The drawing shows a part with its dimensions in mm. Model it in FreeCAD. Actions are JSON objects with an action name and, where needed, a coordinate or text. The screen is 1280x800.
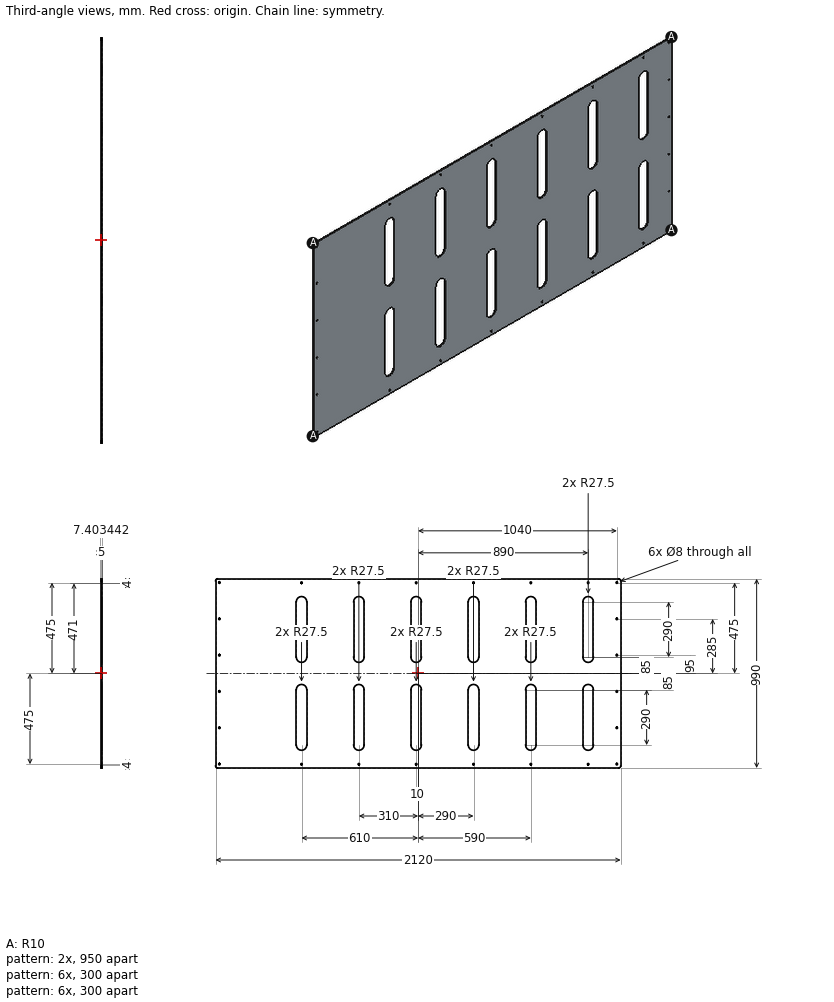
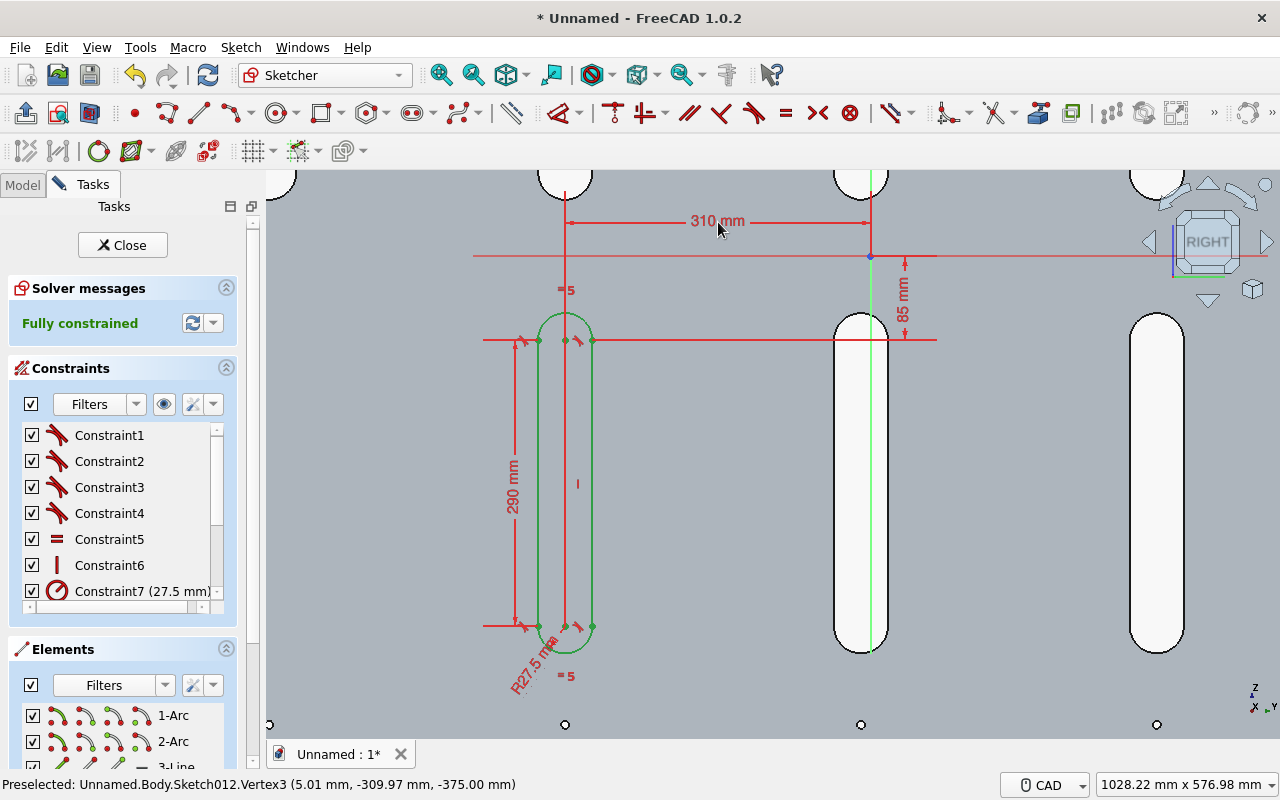
{"action": "left_click", "coordinate": [123, 245]}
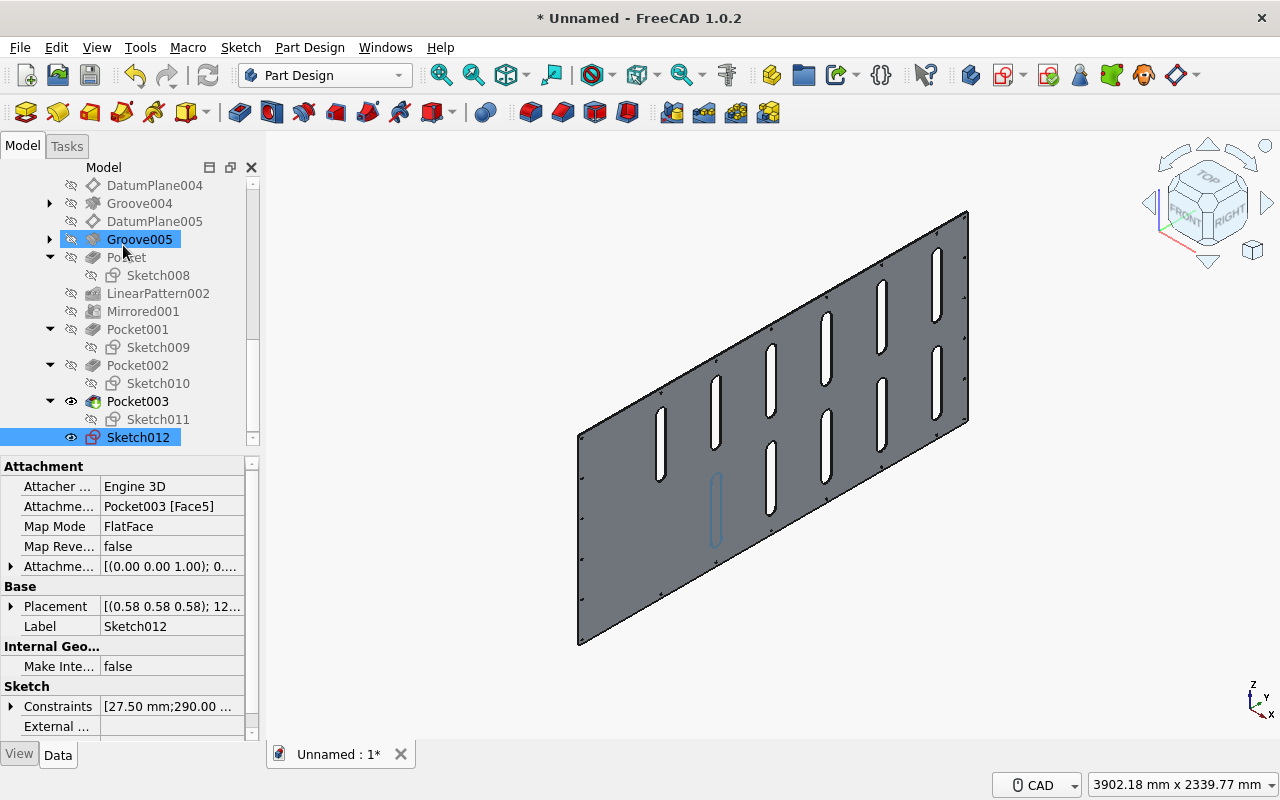
{"action": "left_click", "coordinate": [240, 112]}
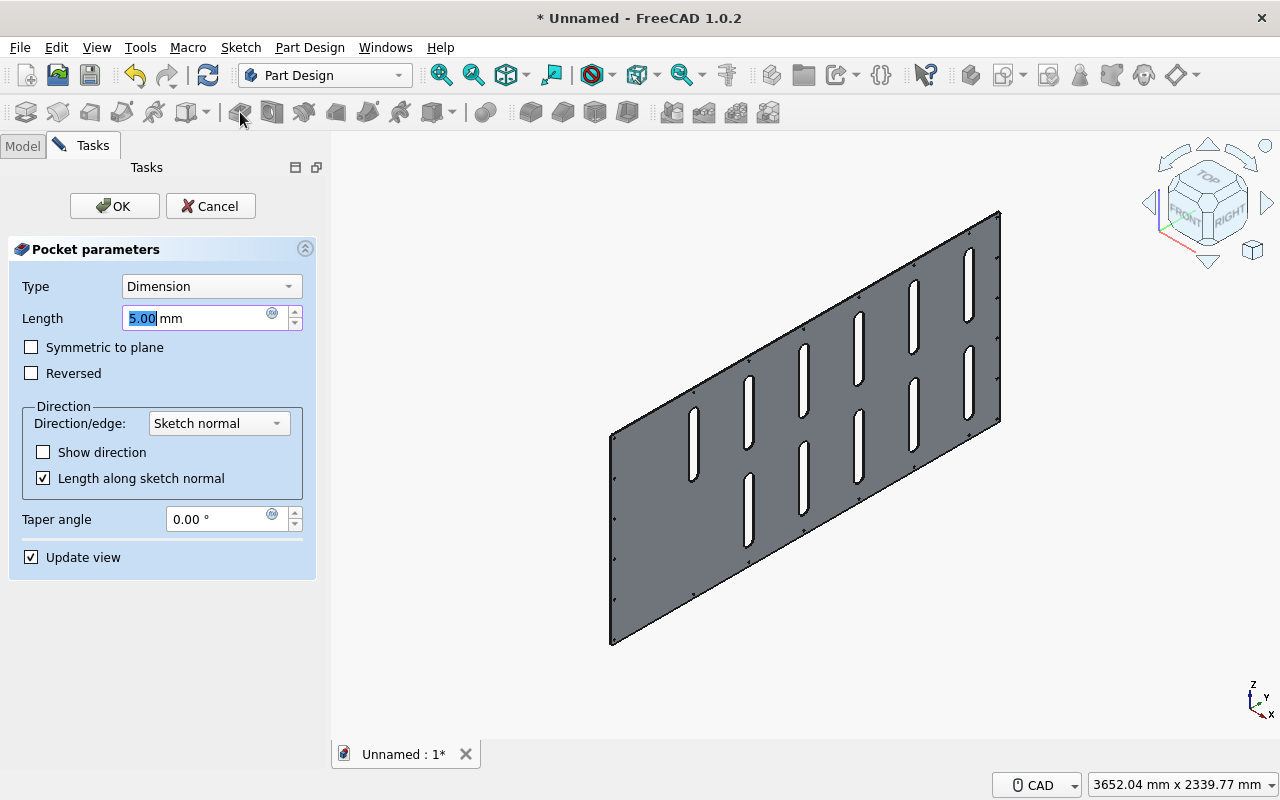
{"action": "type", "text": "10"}
{"action": "key", "text": "Tab"}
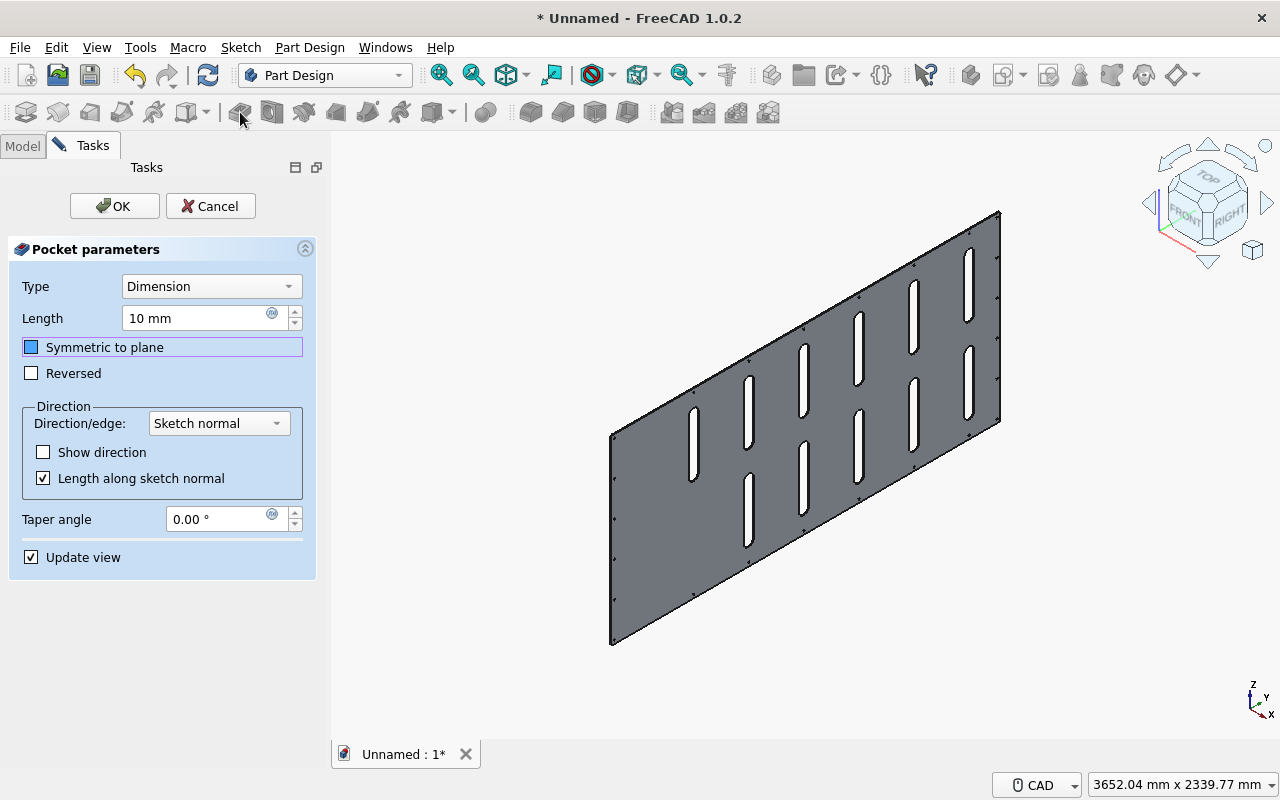
{"action": "left_click", "coordinate": [115, 206]}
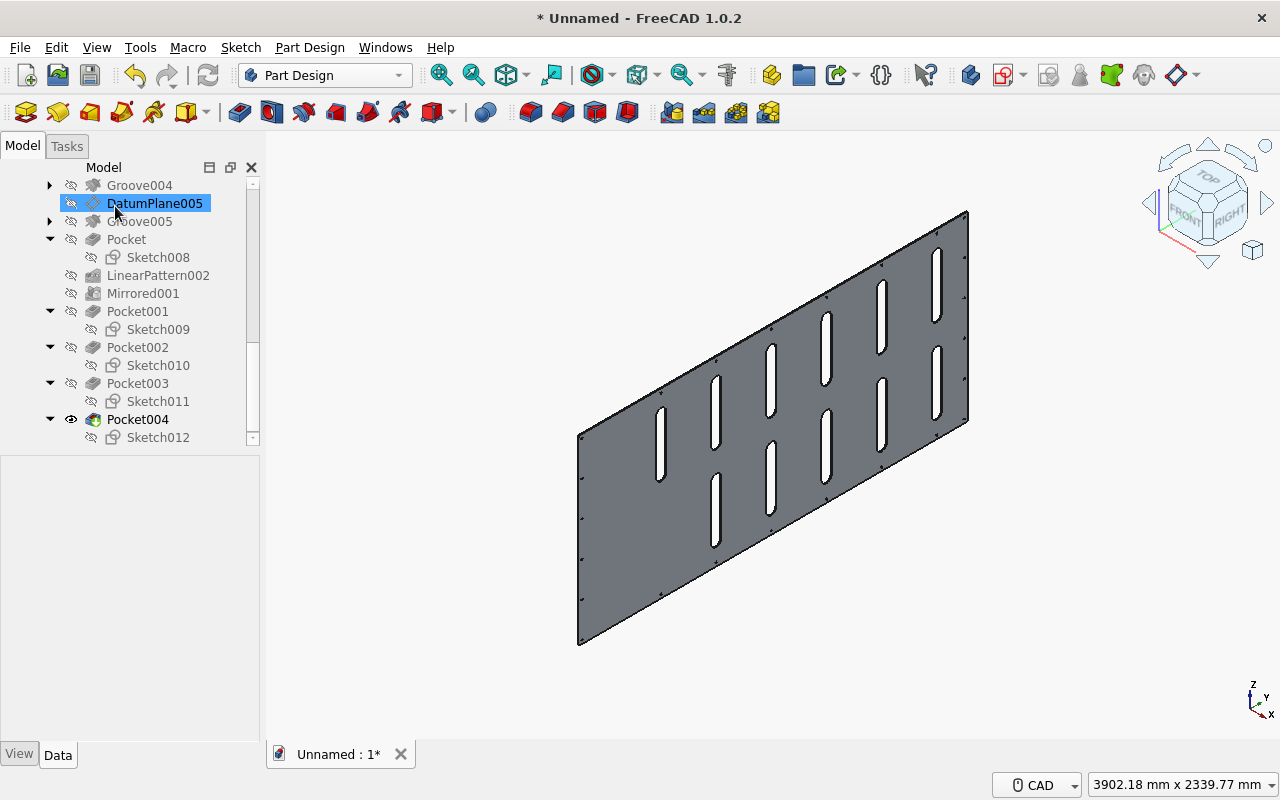
{"action": "left_click", "coordinate": [662, 522]}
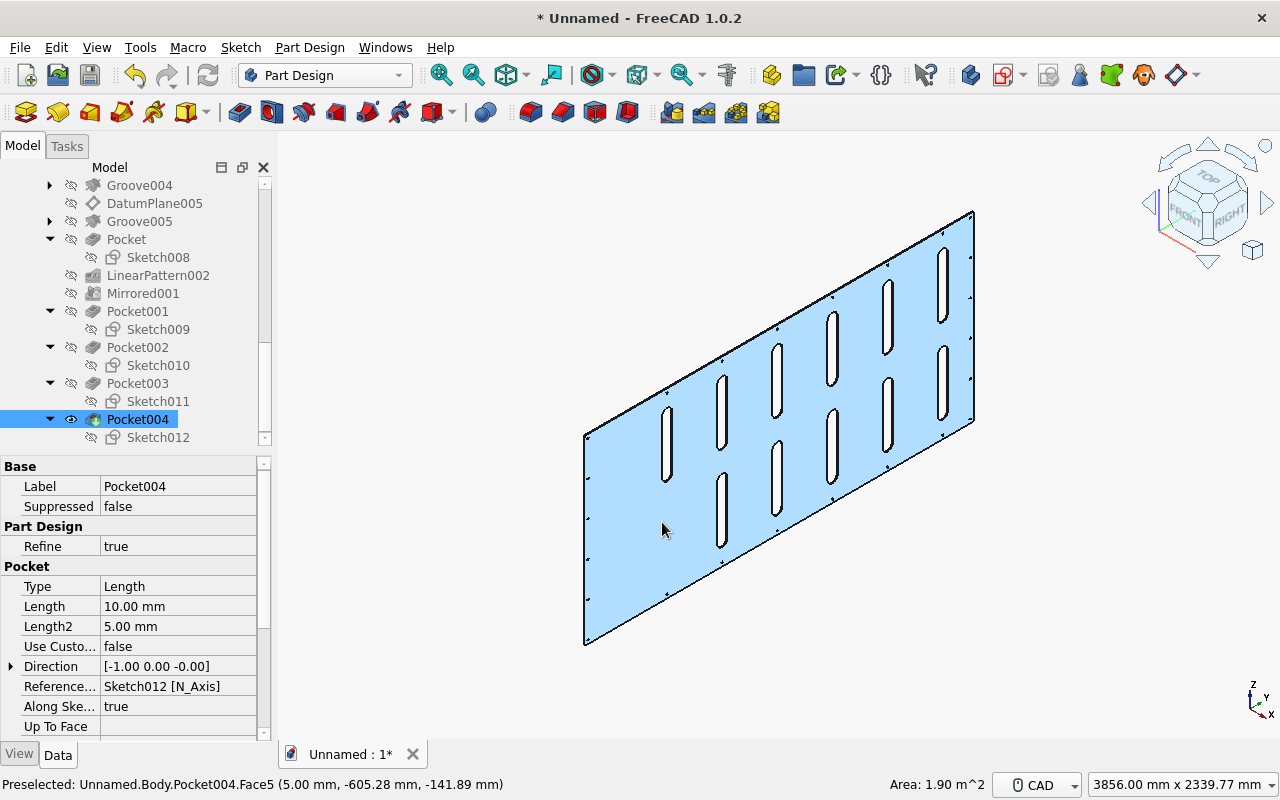
{"action": "left_click", "coordinate": [1004, 76]}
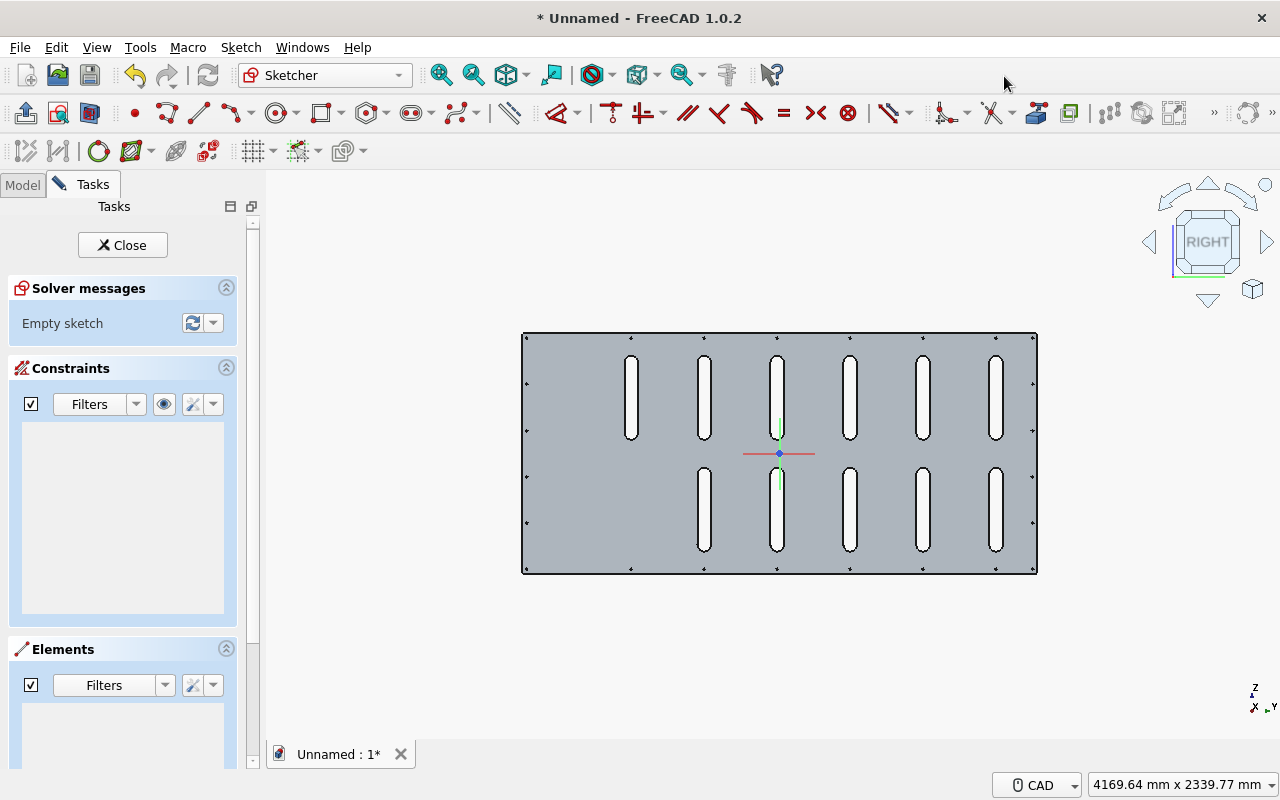
{"action": "scroll", "coordinate": [701, 518], "scroll_direction": "up", "scroll_amount": 7}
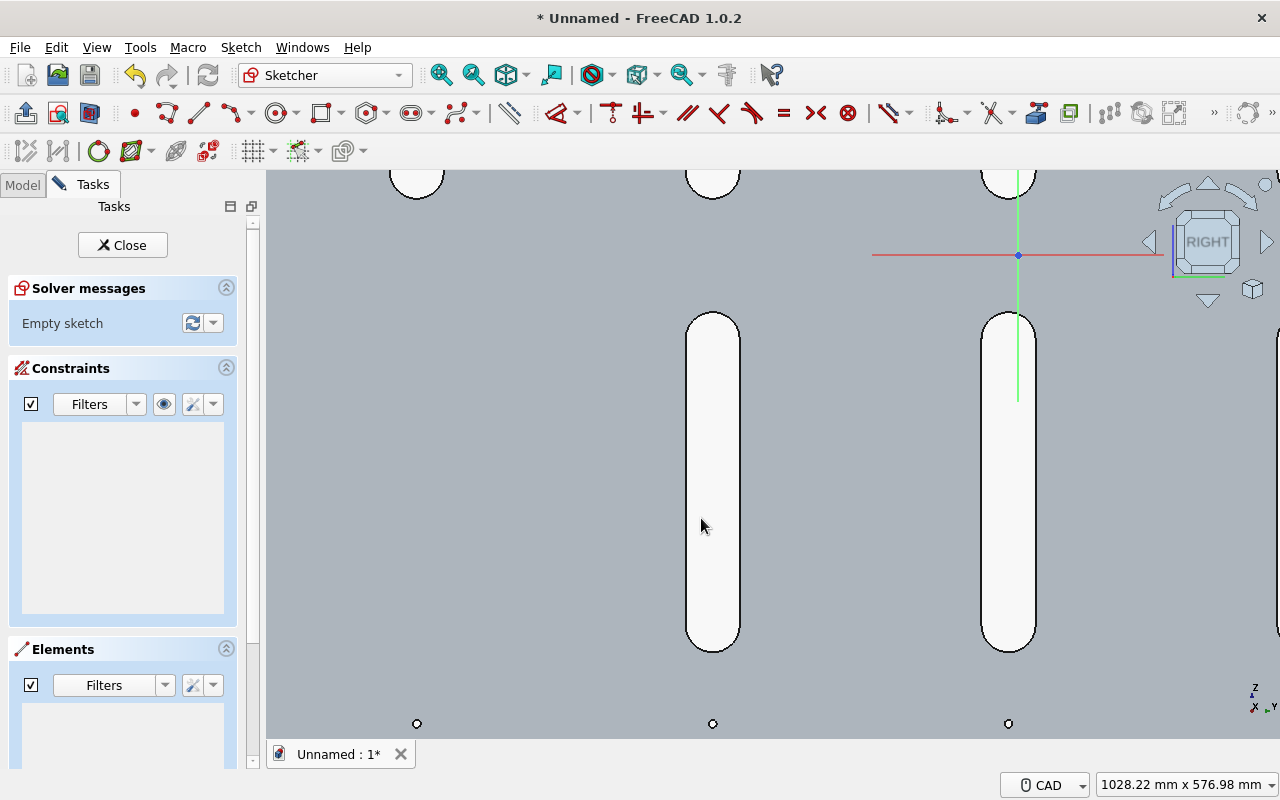
{"action": "left_click", "coordinate": [412, 114]}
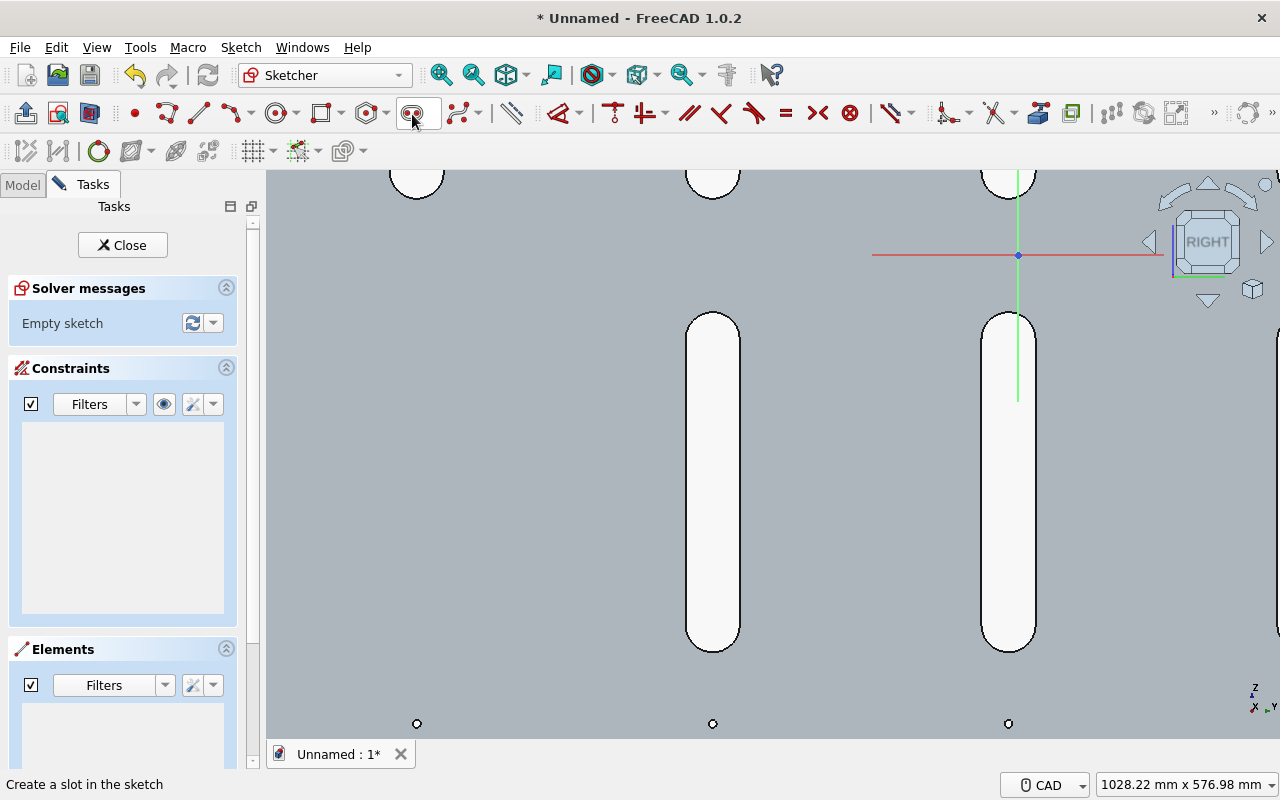
{"action": "left_click", "coordinate": [417, 625]}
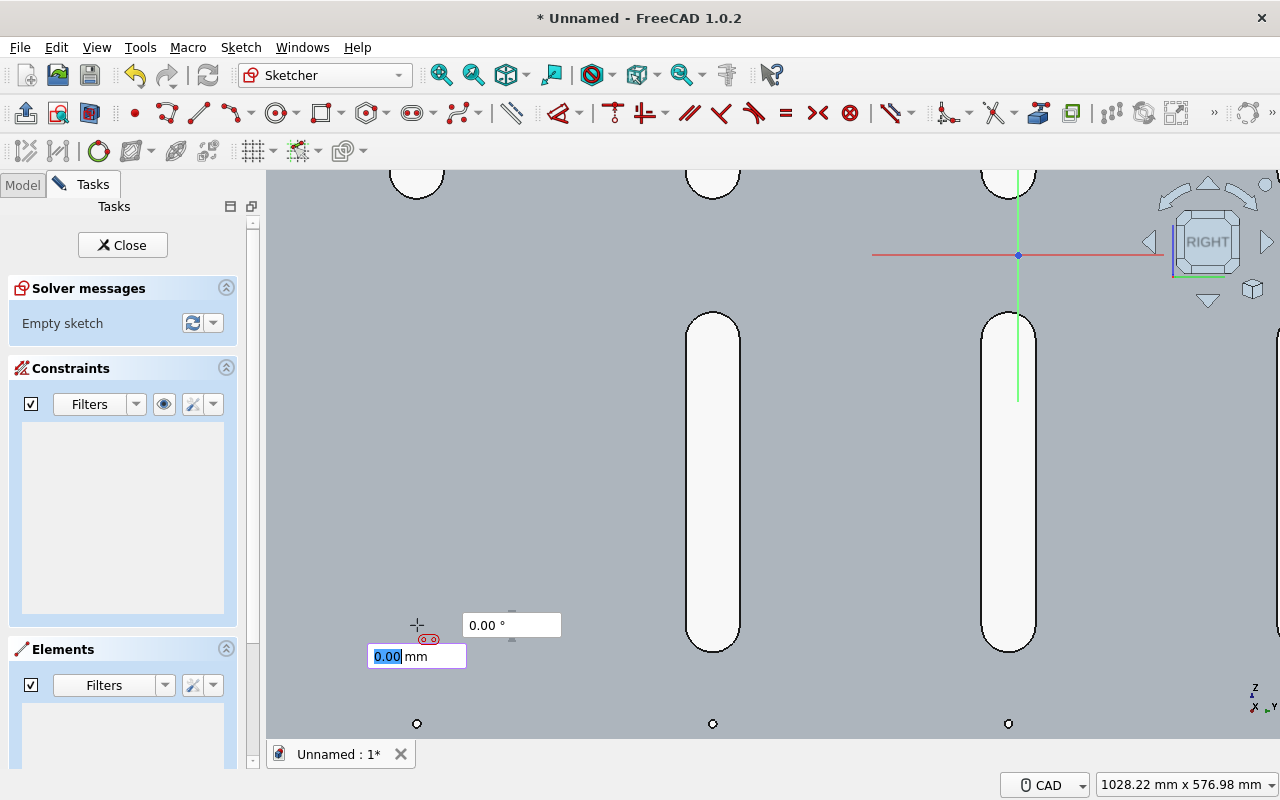
{"action": "left_click", "coordinate": [417, 339]}